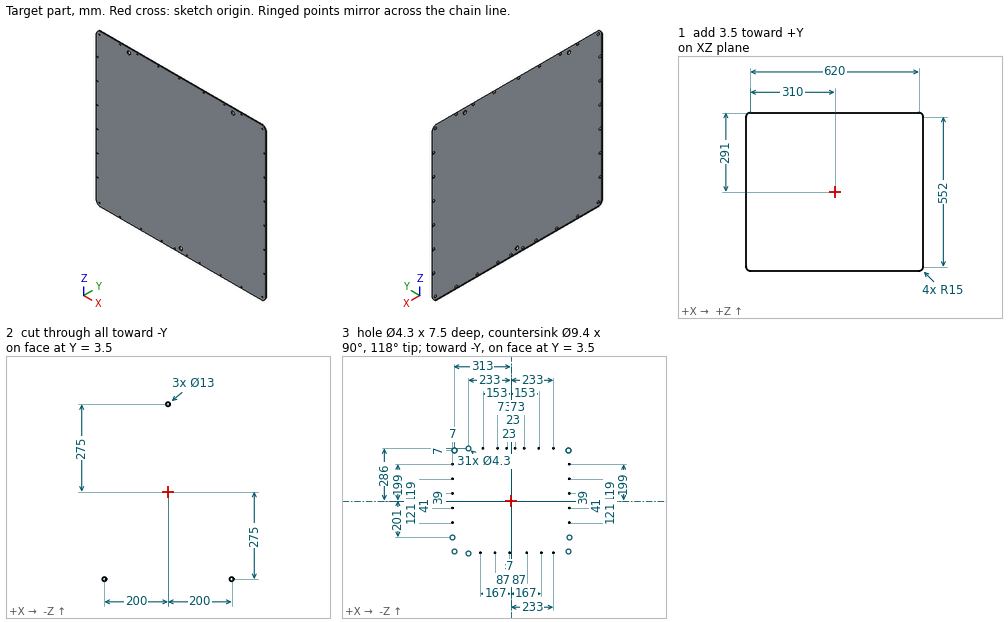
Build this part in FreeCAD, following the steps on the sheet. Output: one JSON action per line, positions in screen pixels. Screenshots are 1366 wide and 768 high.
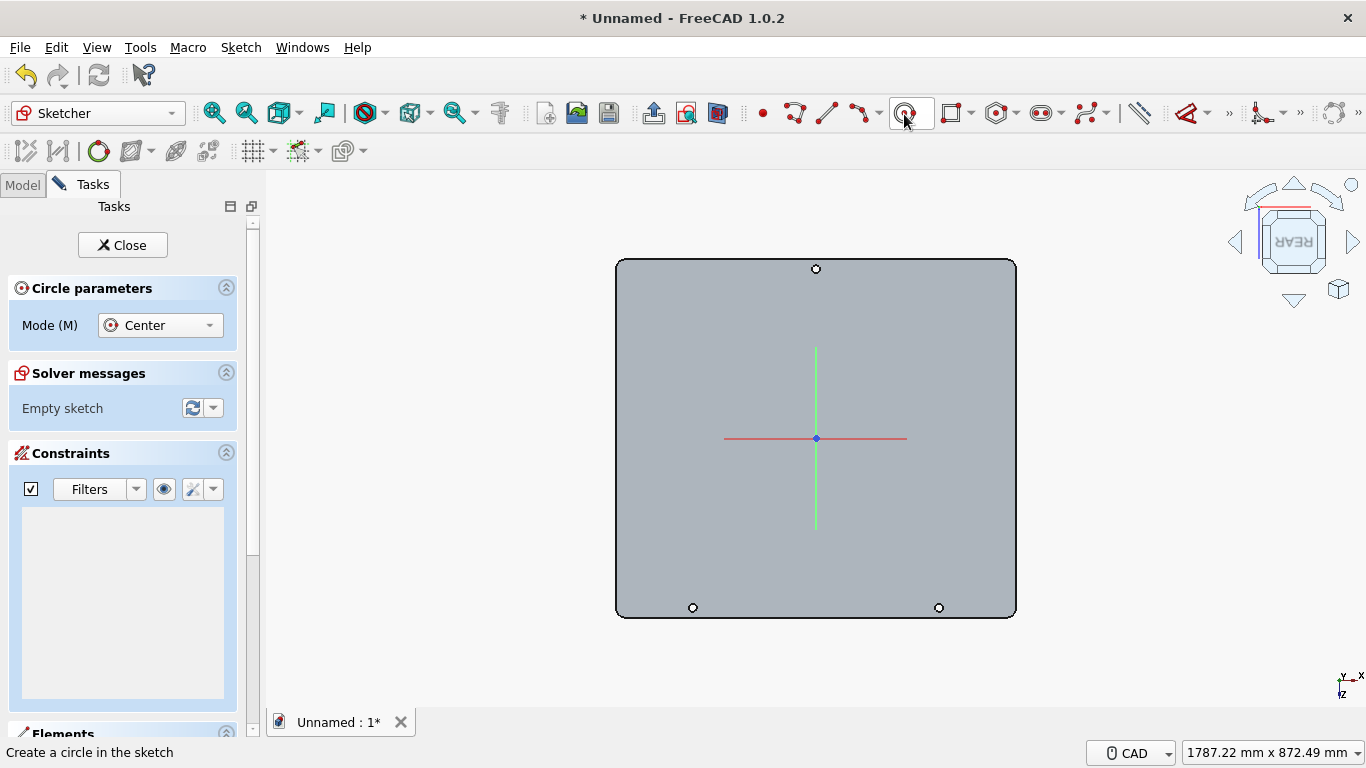
{"action": "scroll", "coordinate": [673, 262], "scroll_direction": "up", "scroll_amount": 15}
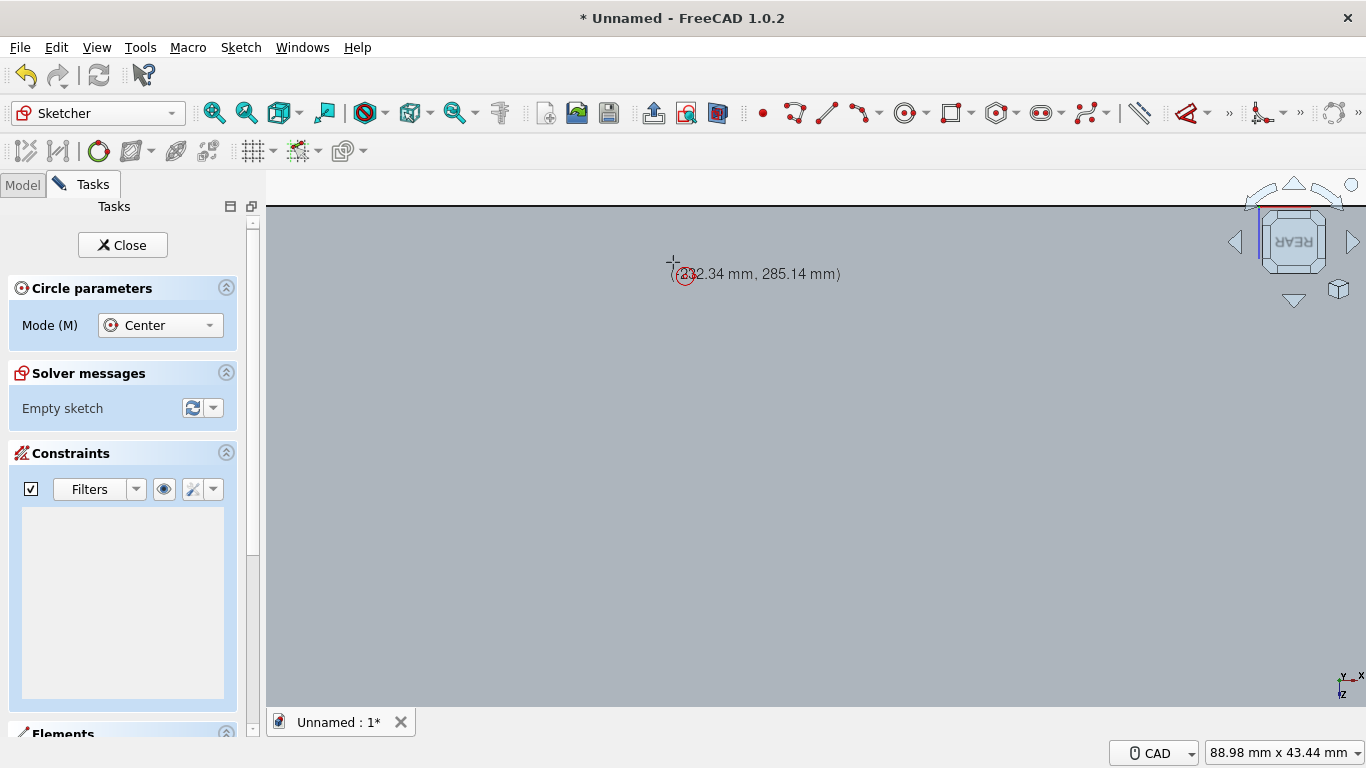
{"action": "scroll", "coordinate": [601, 262], "scroll_direction": "down", "scroll_amount": 15}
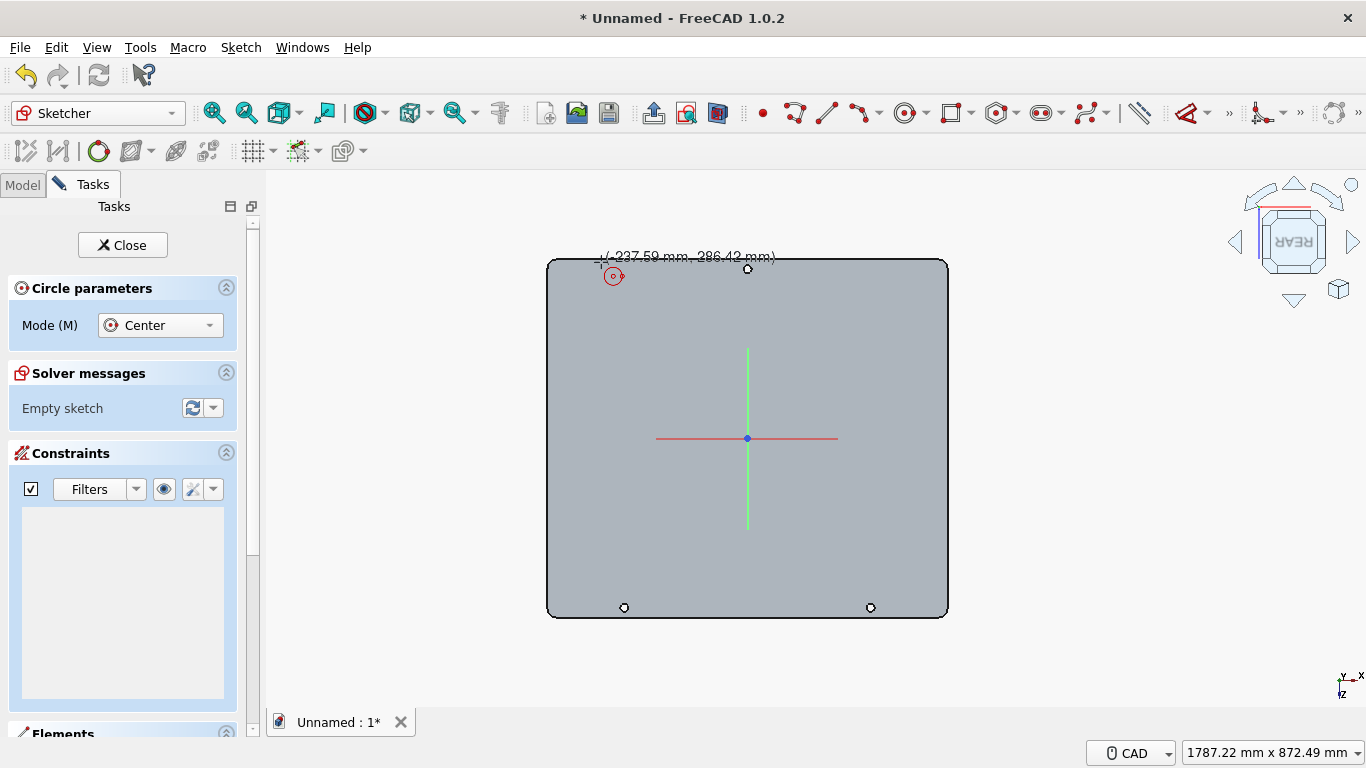
{"action": "left_click", "coordinate": [604, 262]}
{"action": "mouse_move", "coordinate": [605, 262]}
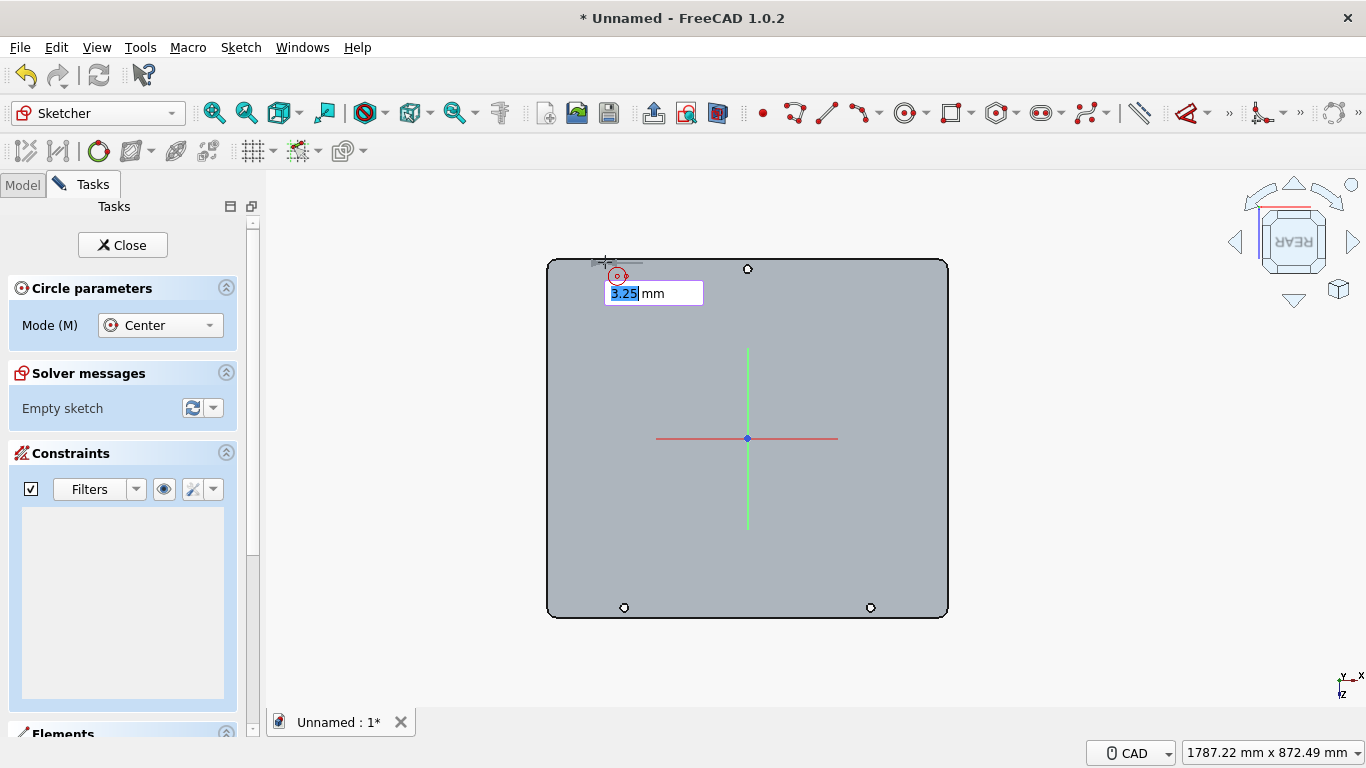
{"action": "type", "text": "4.3"}
{"action": "key", "text": "Return"}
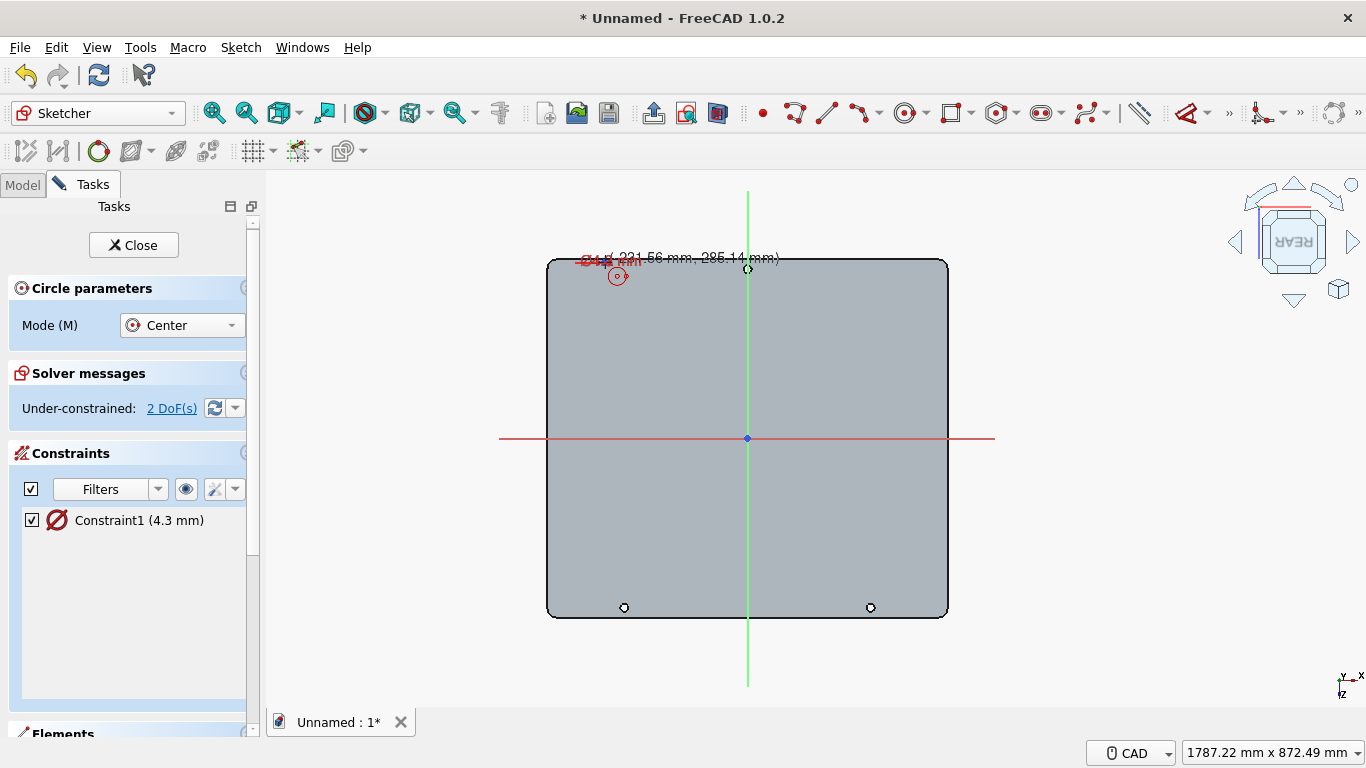
{"action": "scroll", "coordinate": [555, 267], "scroll_direction": "up", "scroll_amount": 15}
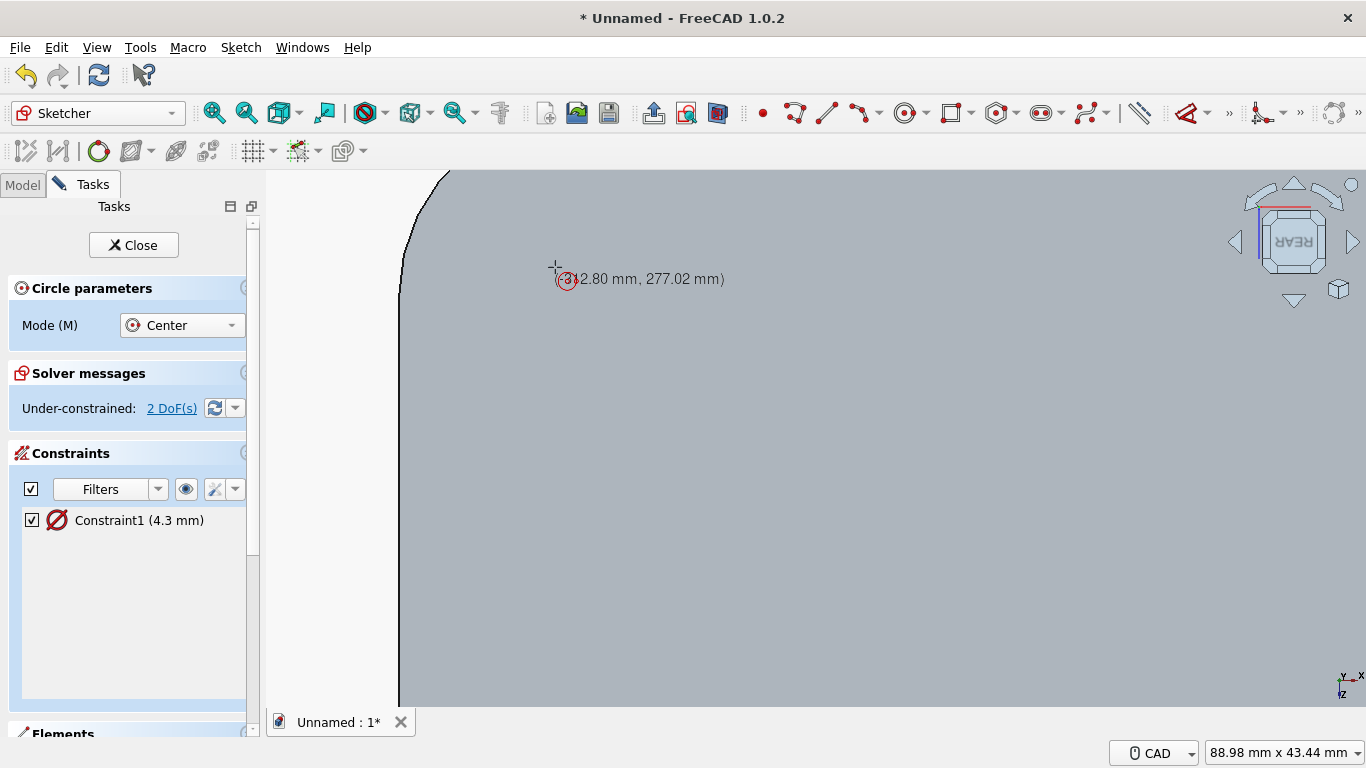
{"action": "scroll", "coordinate": [555, 267], "scroll_direction": "down", "scroll_amount": 15}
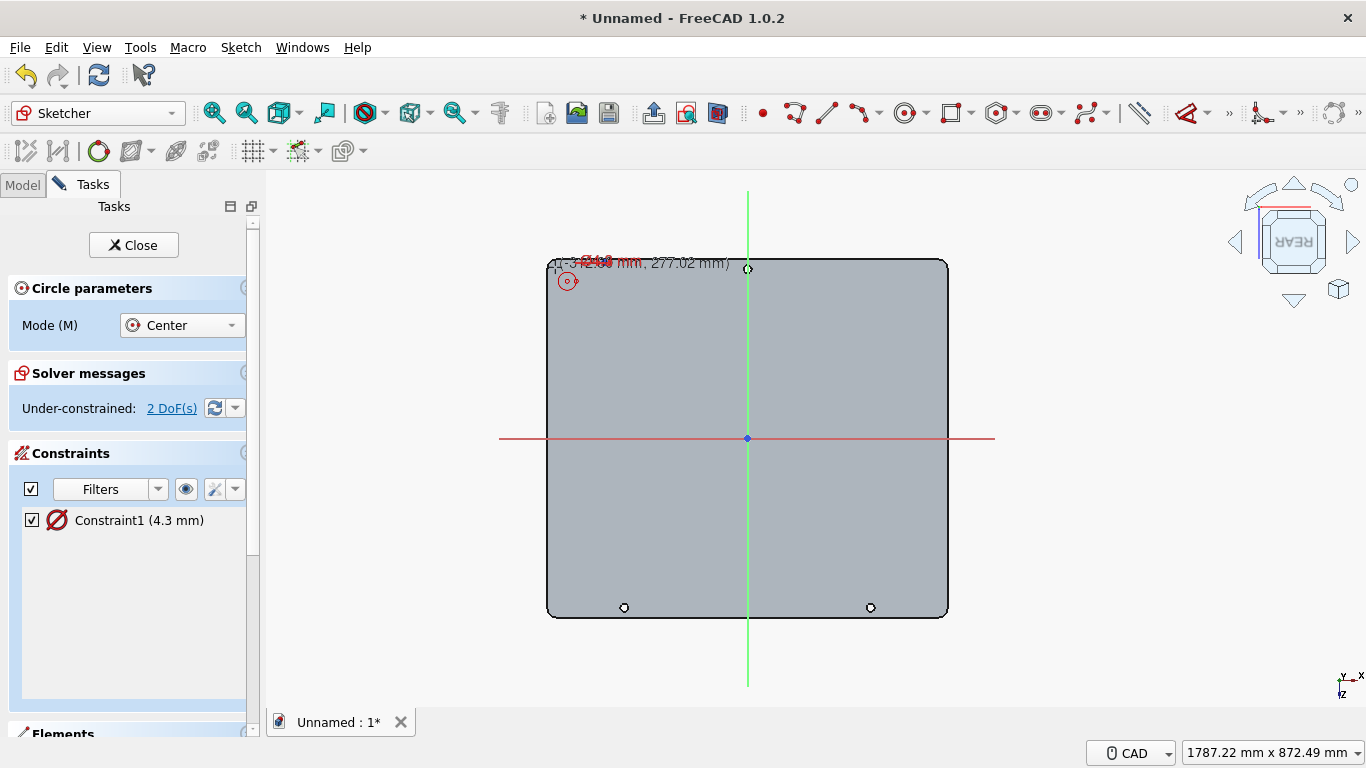
{"action": "left_click", "coordinate": [555, 267]}
{"action": "mouse_move", "coordinate": [556, 266]}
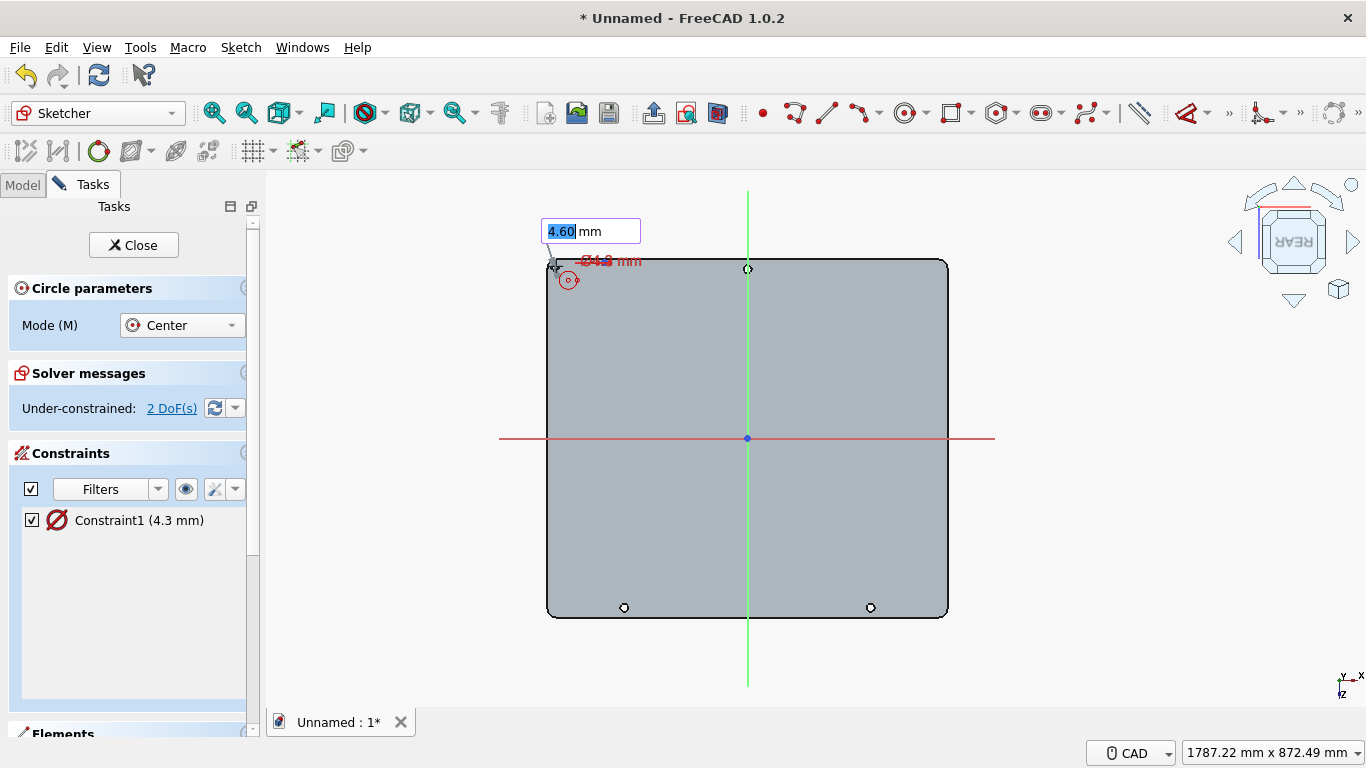
{"action": "type", "text": "4.3"}
{"action": "key", "text": "Return"}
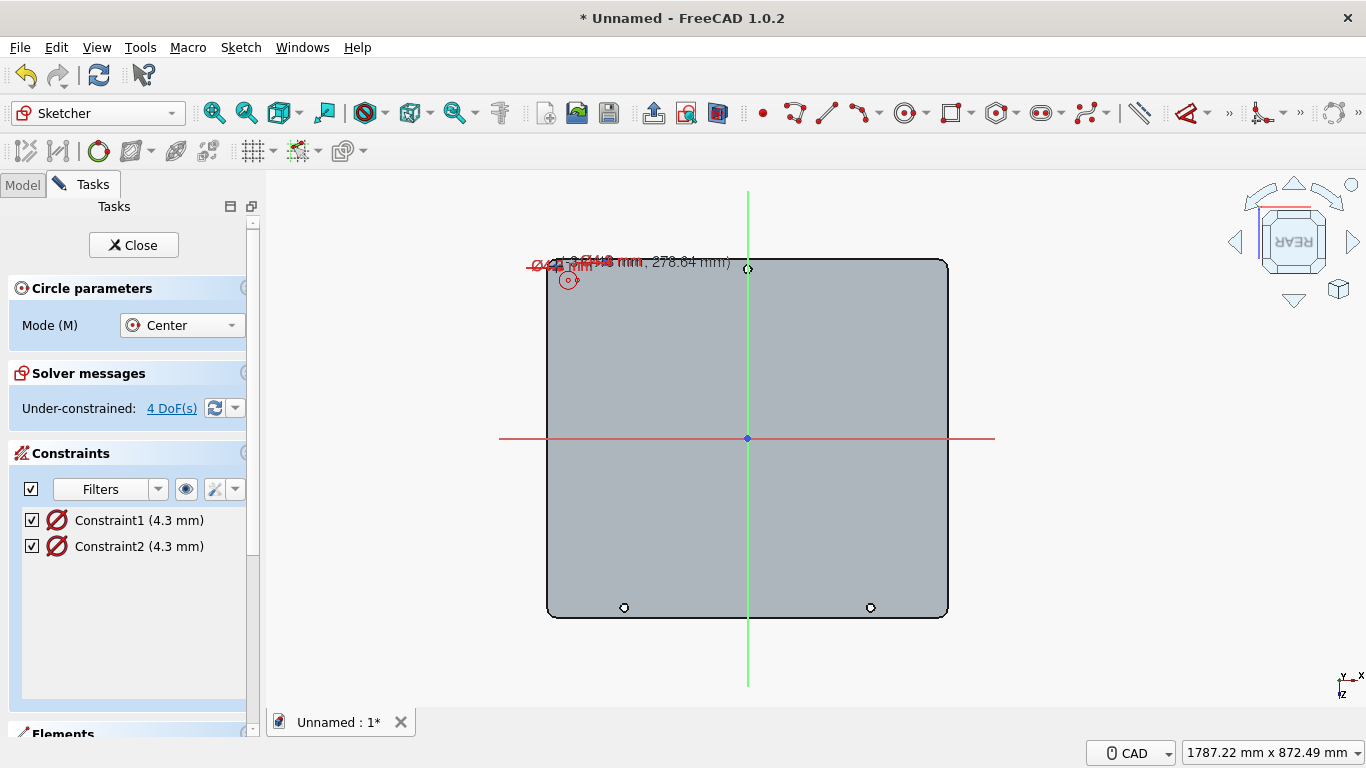
{"action": "scroll", "coordinate": [653, 262], "scroll_direction": "up", "scroll_amount": 15}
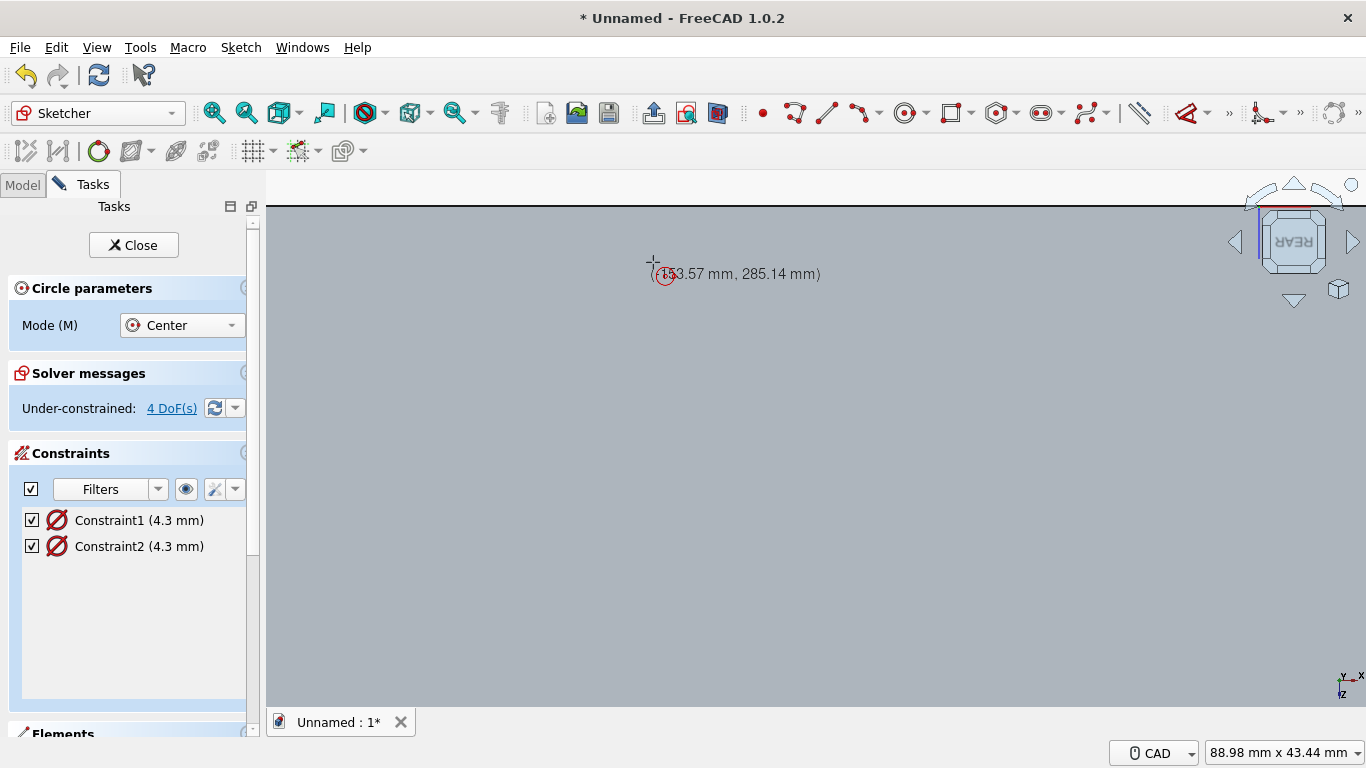
{"action": "scroll", "coordinate": [653, 262], "scroll_direction": "down", "scroll_amount": 15}